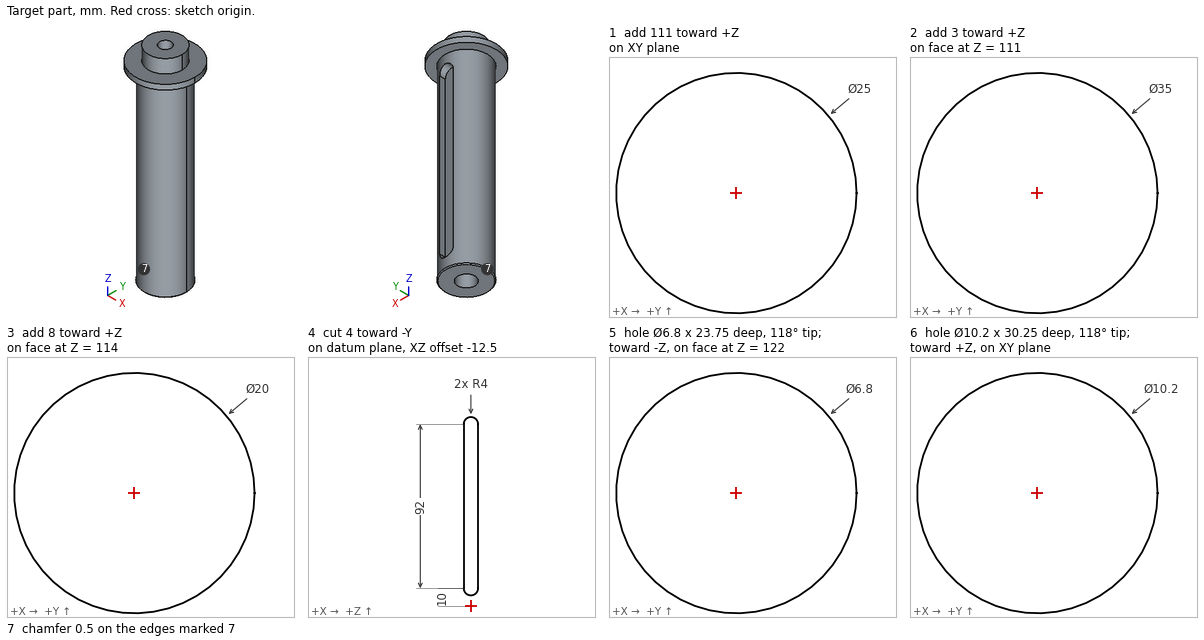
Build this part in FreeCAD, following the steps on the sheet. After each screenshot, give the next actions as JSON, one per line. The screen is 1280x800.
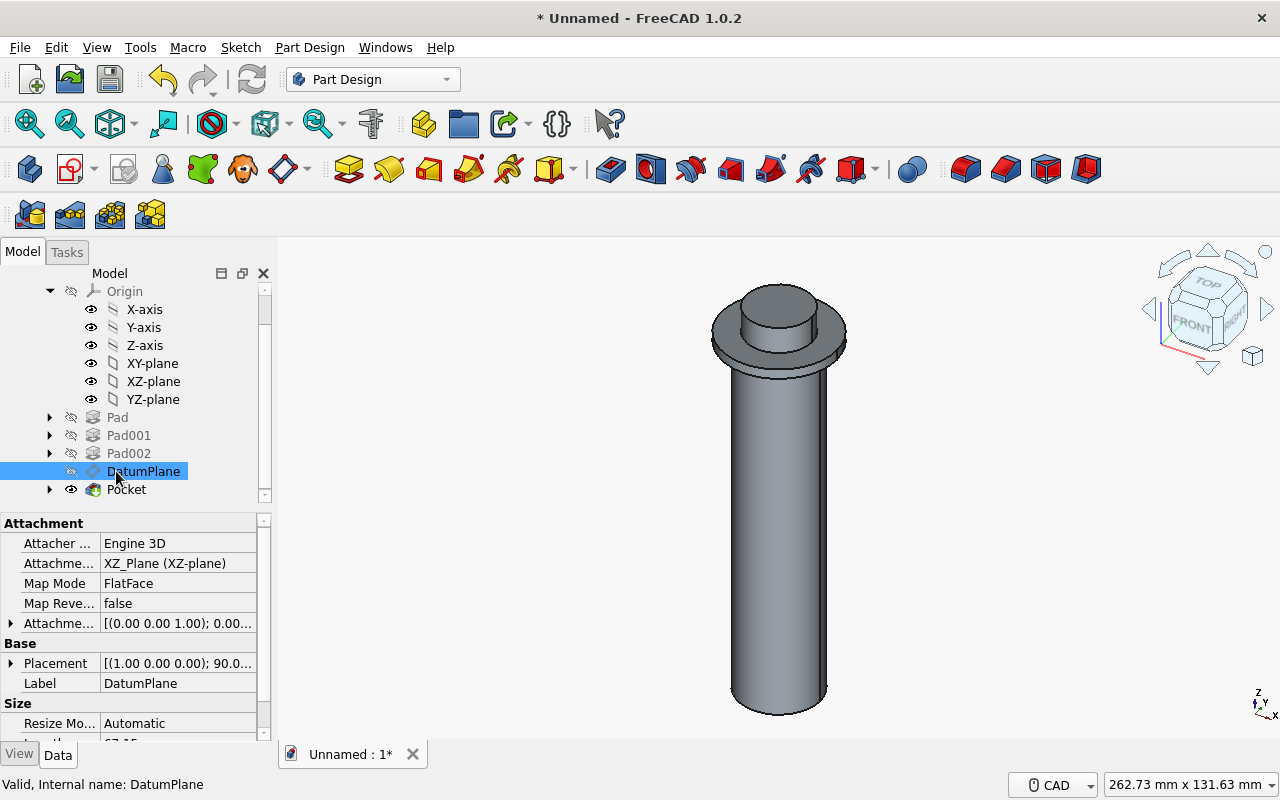
{"action": "left_click", "coordinate": [779, 305]}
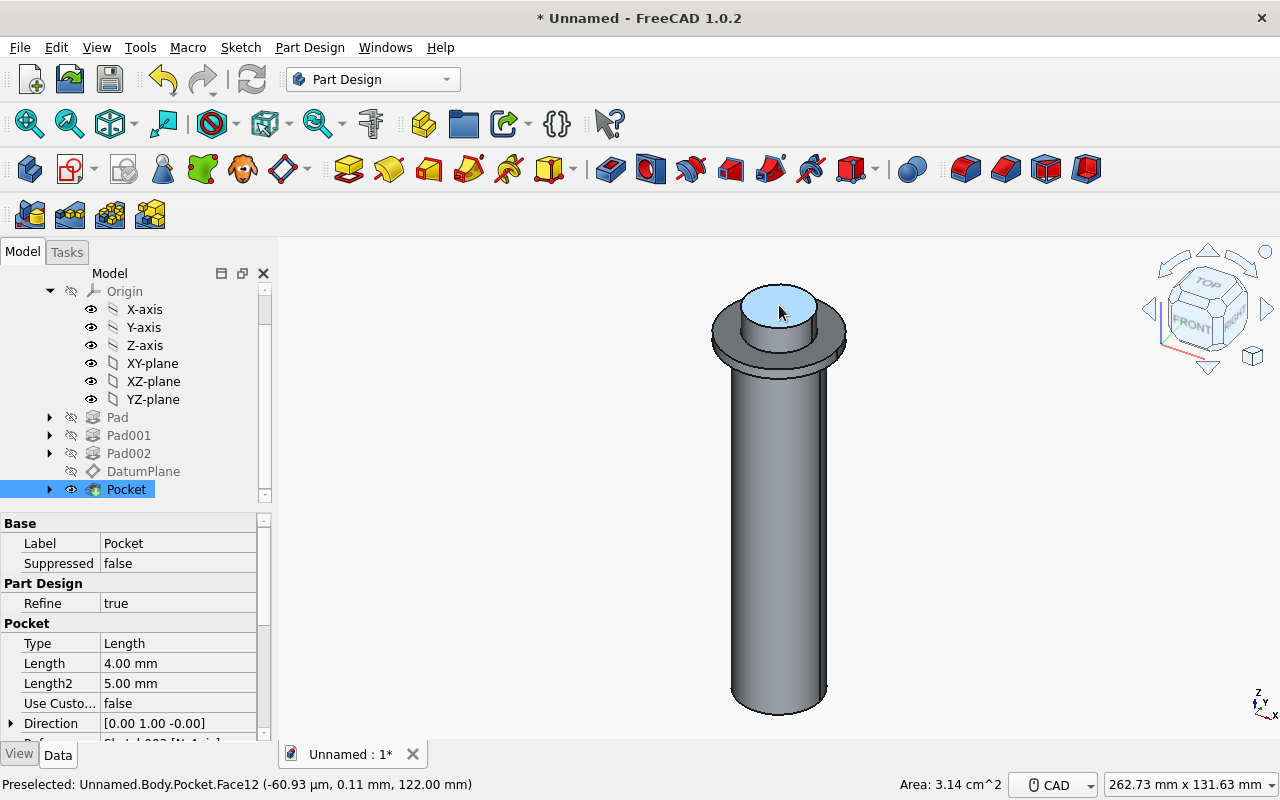
{"action": "left_click", "coordinate": [70, 170]}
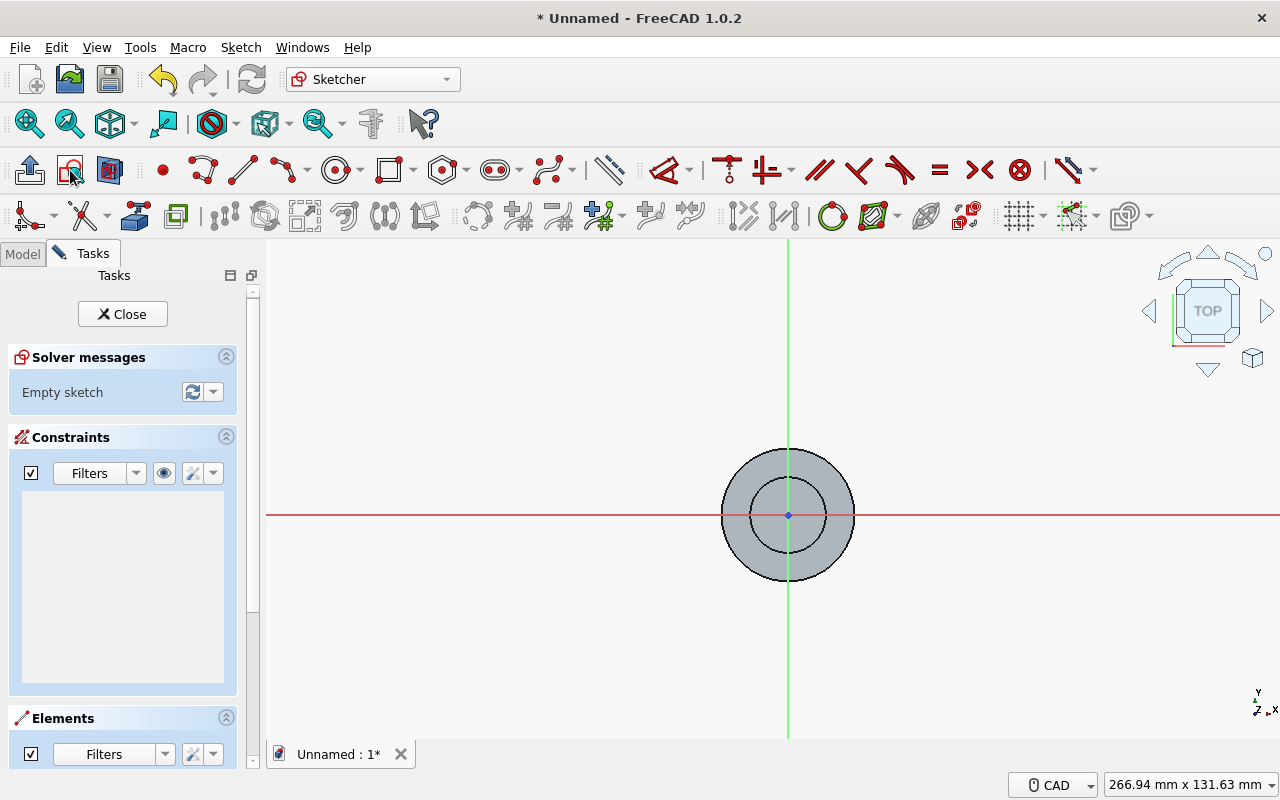
{"action": "scroll", "coordinate": [796, 518], "scroll_direction": "up", "scroll_amount": 12}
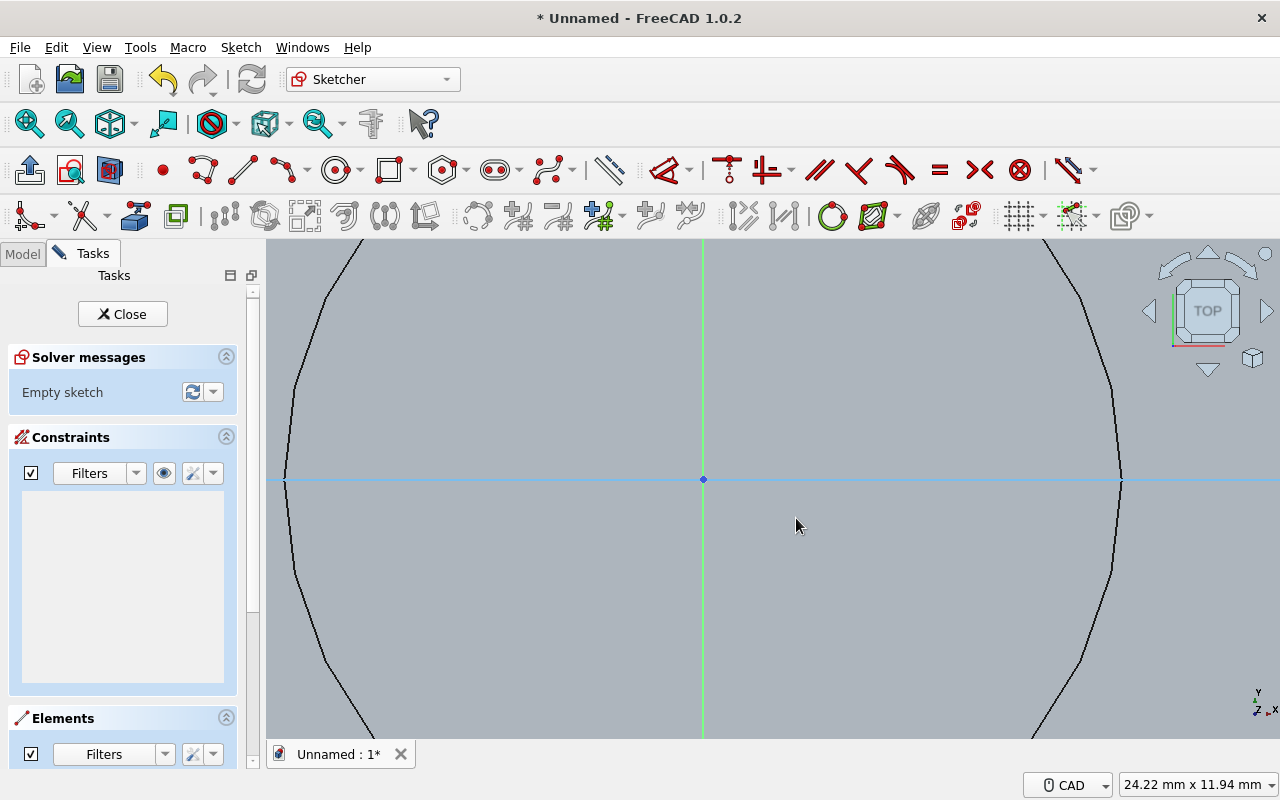
{"action": "left_click", "coordinate": [336, 170]}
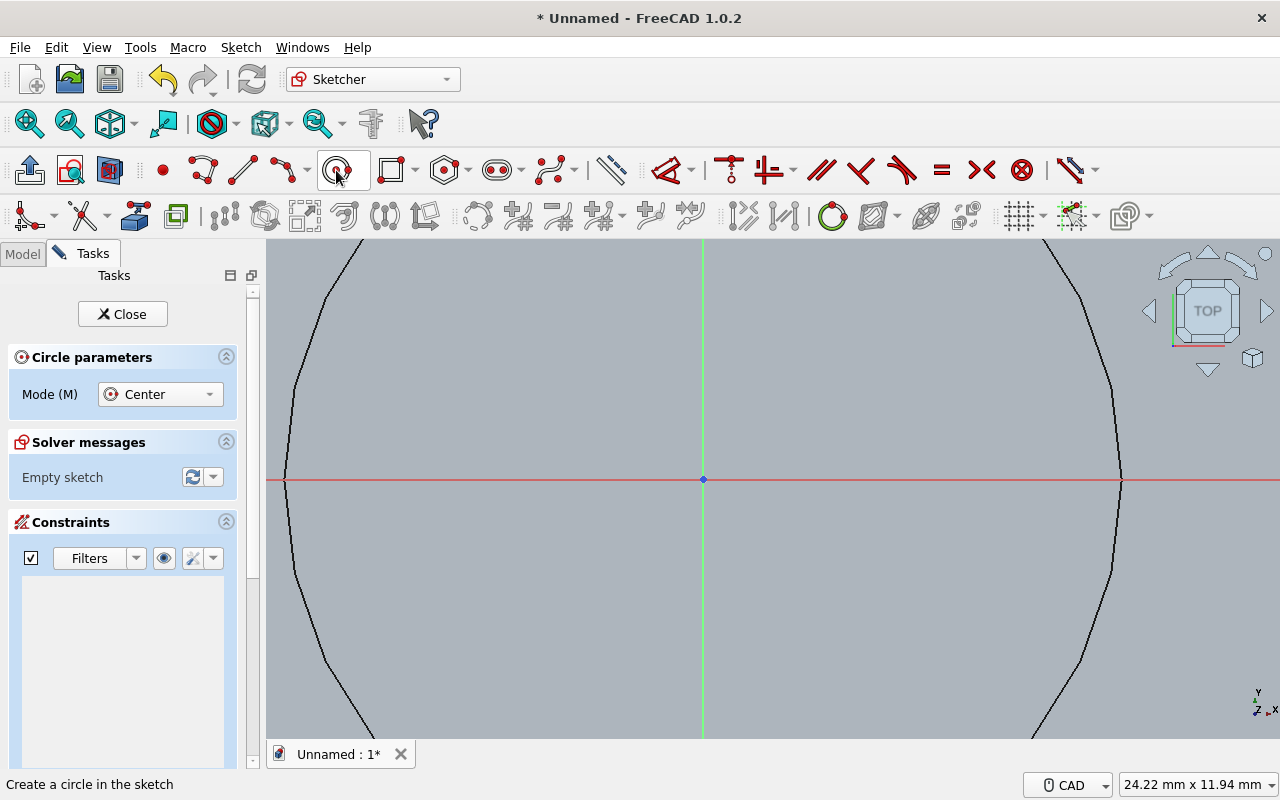
{"action": "left_click", "coordinate": [703, 480]}
{"action": "mouse_move", "coordinate": [804, 379]}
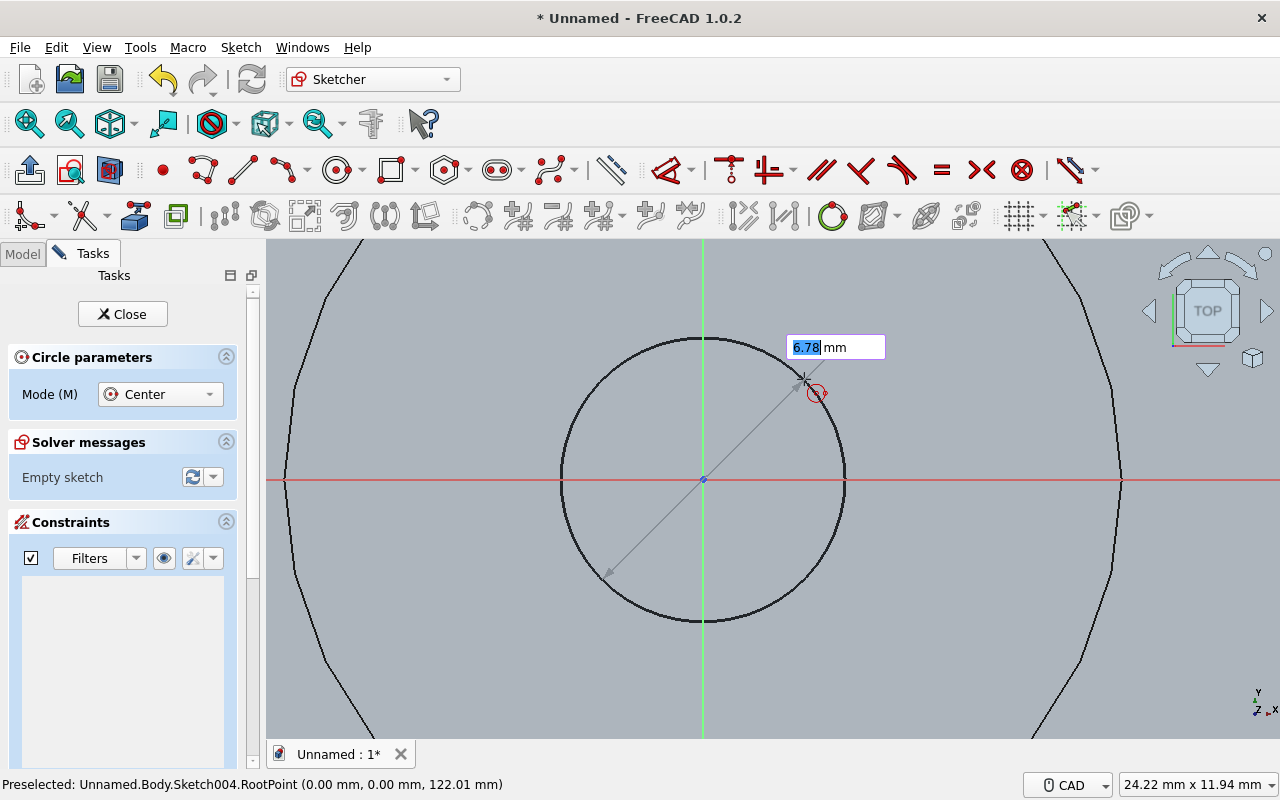
{"action": "type", "text": "6.8"}
{"action": "key", "text": "Return"}
{"action": "key", "text": "Escape"}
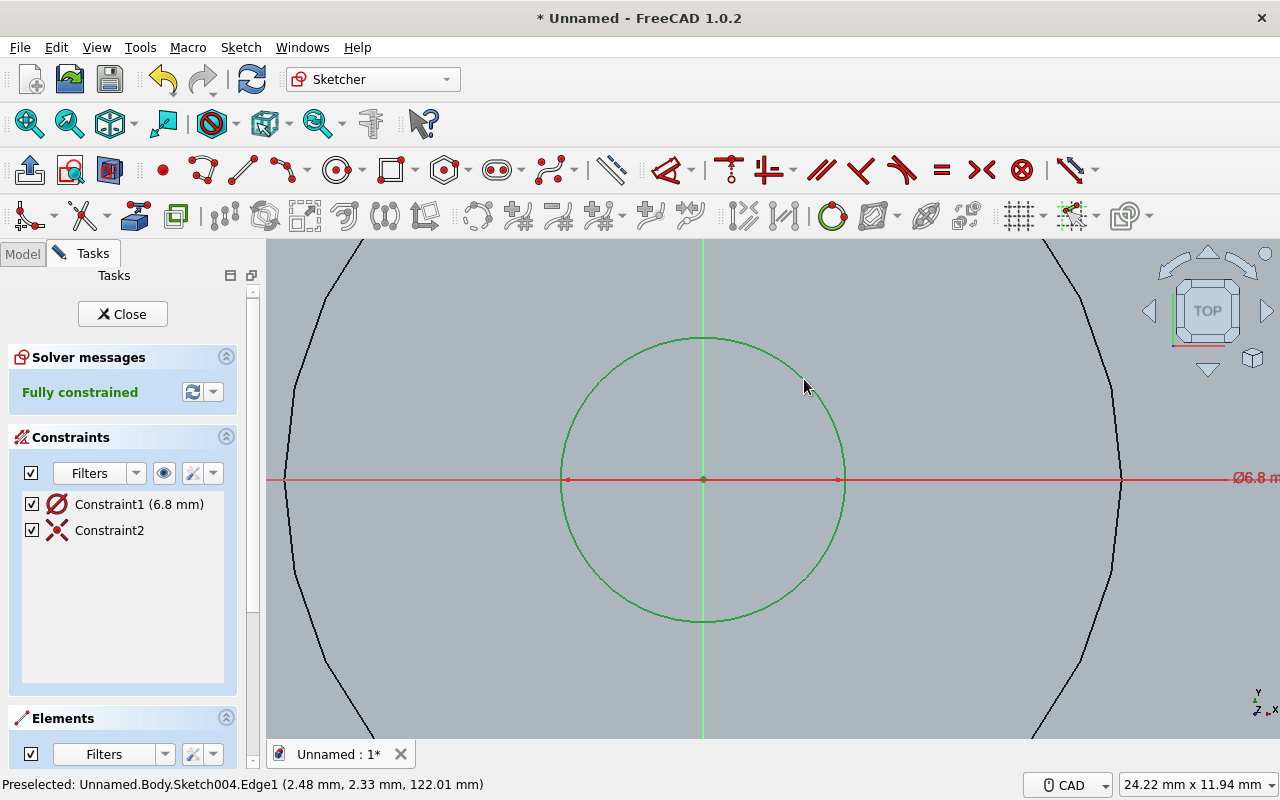
{"action": "left_click", "coordinate": [123, 314]}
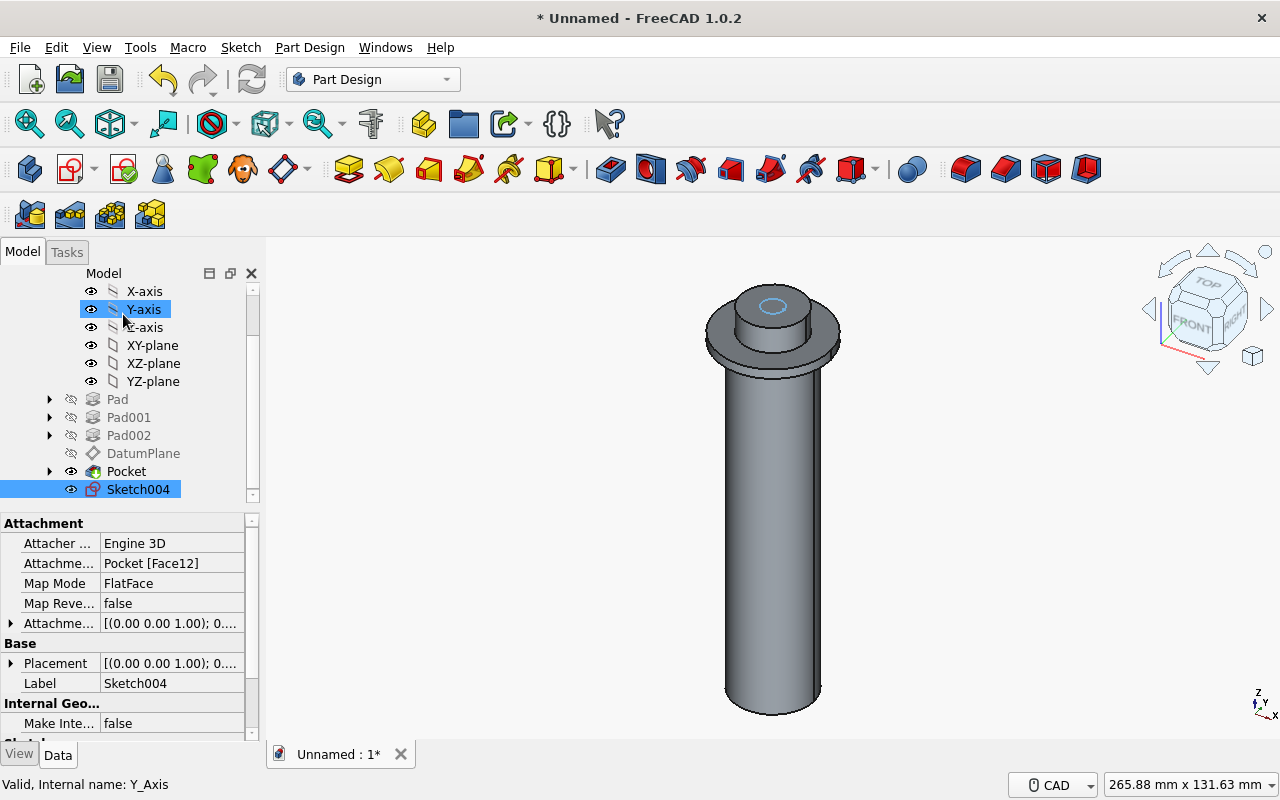
{"action": "left_click", "coordinate": [652, 170]}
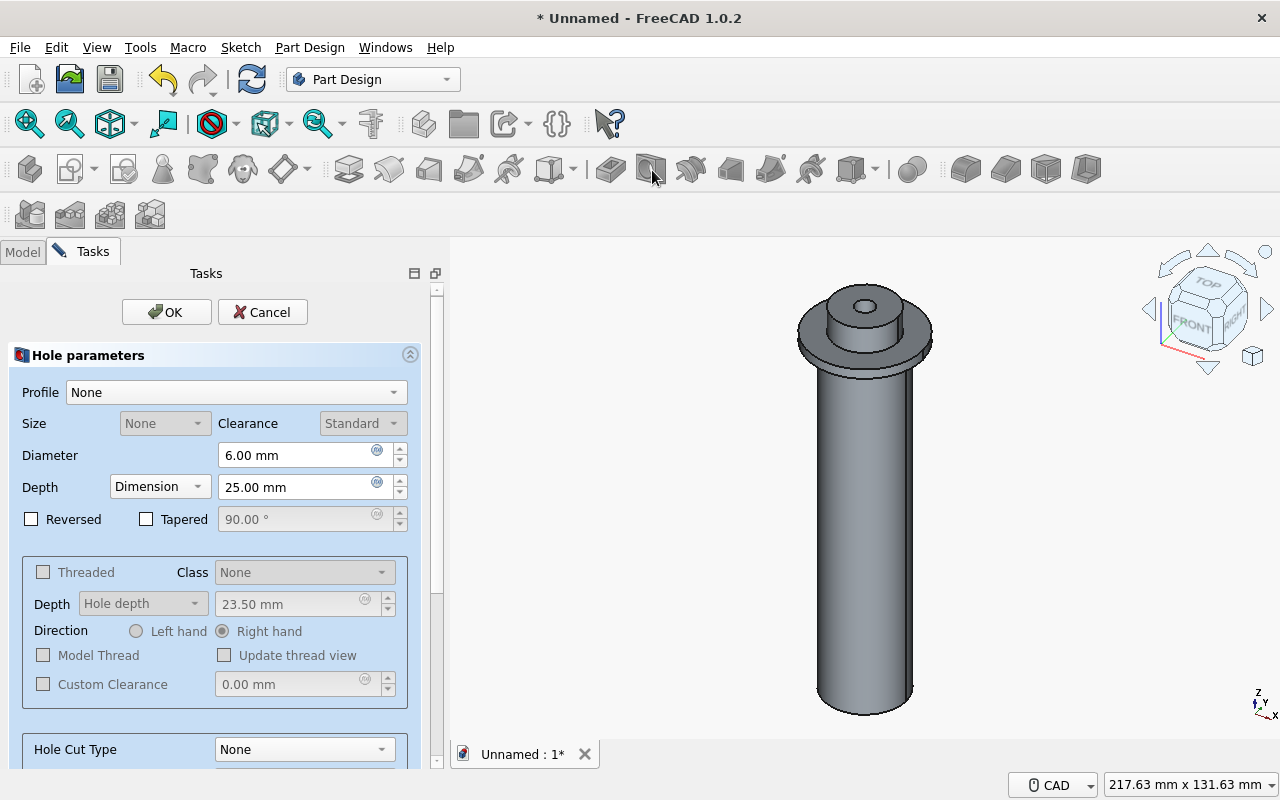
{"action": "triple_click", "coordinate": [305, 455]}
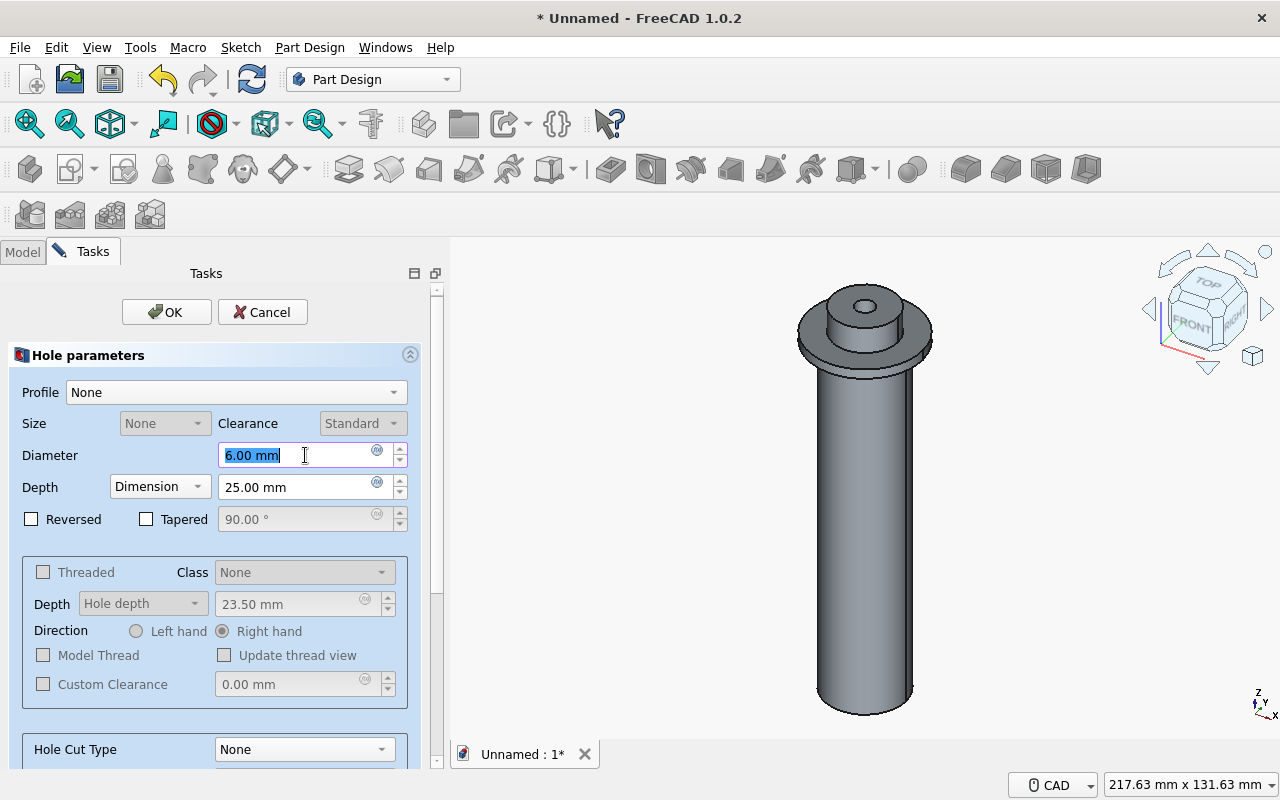
{"action": "type", "text": "6.8"}
{"action": "key", "text": "Tab"}